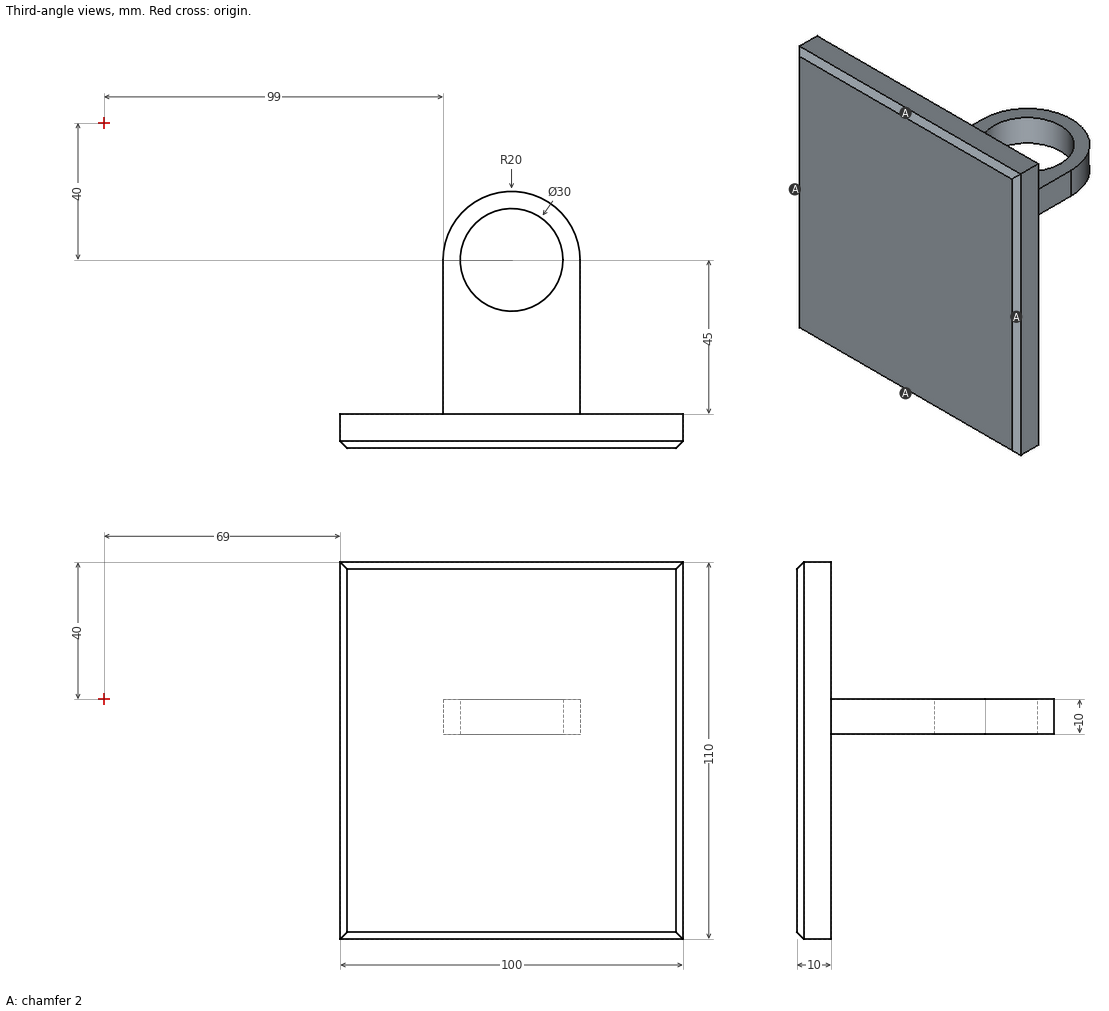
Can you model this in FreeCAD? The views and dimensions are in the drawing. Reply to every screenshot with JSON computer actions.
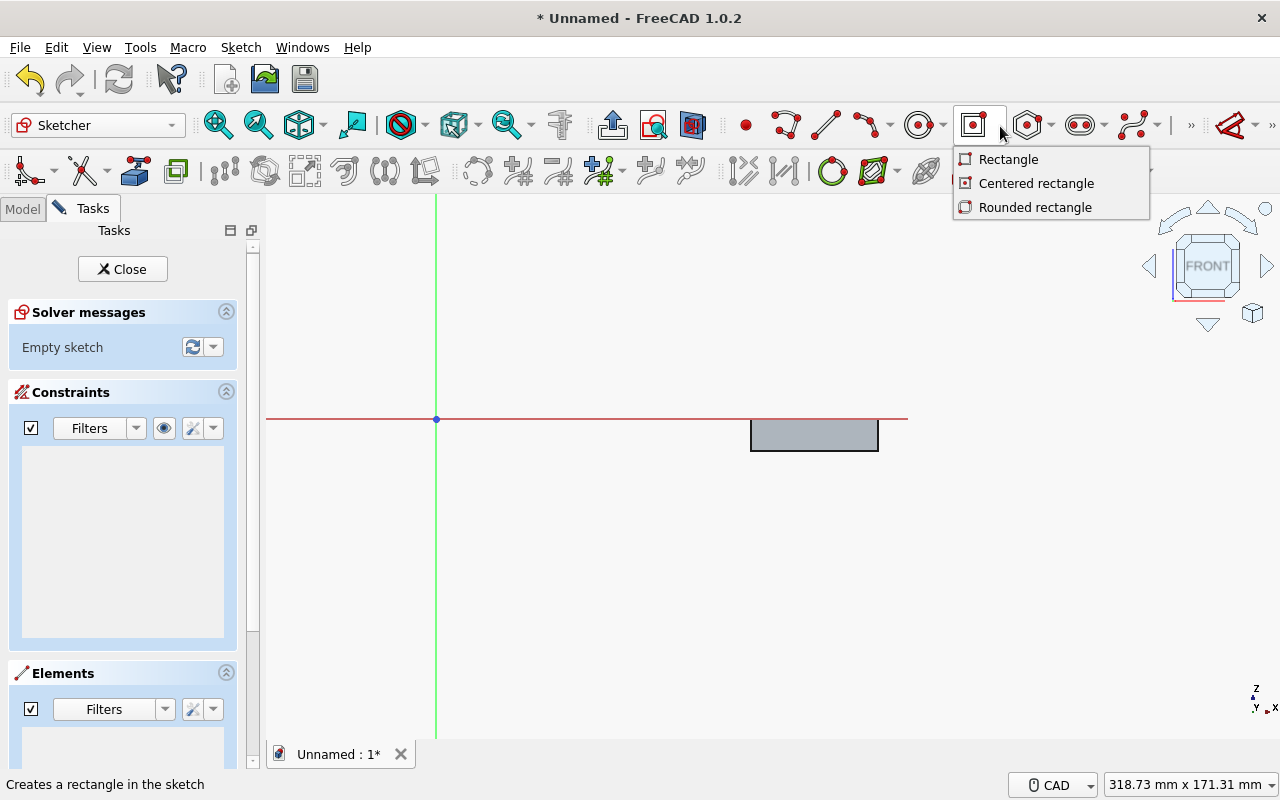
{"action": "left_click", "coordinate": [1052, 159]}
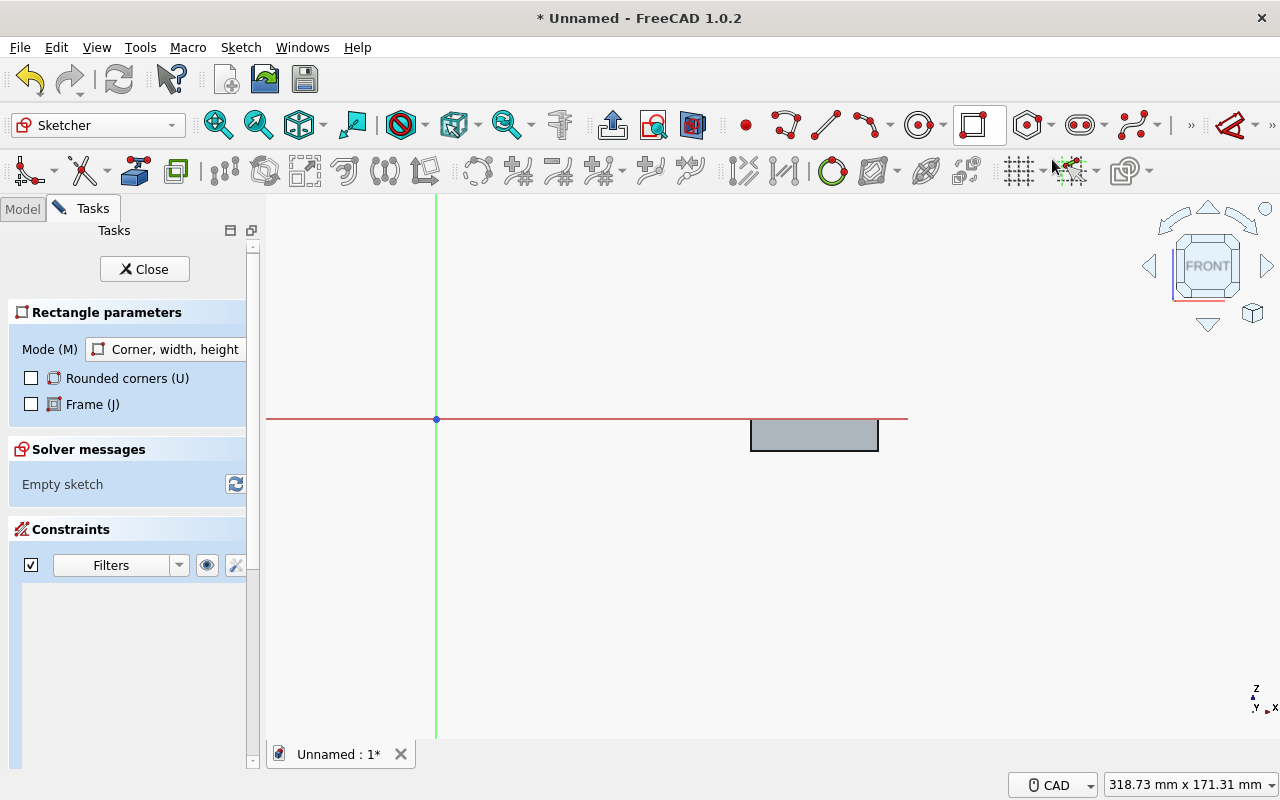
{"action": "left_click", "coordinate": [656, 292]}
{"action": "mouse_move", "coordinate": [974, 642]}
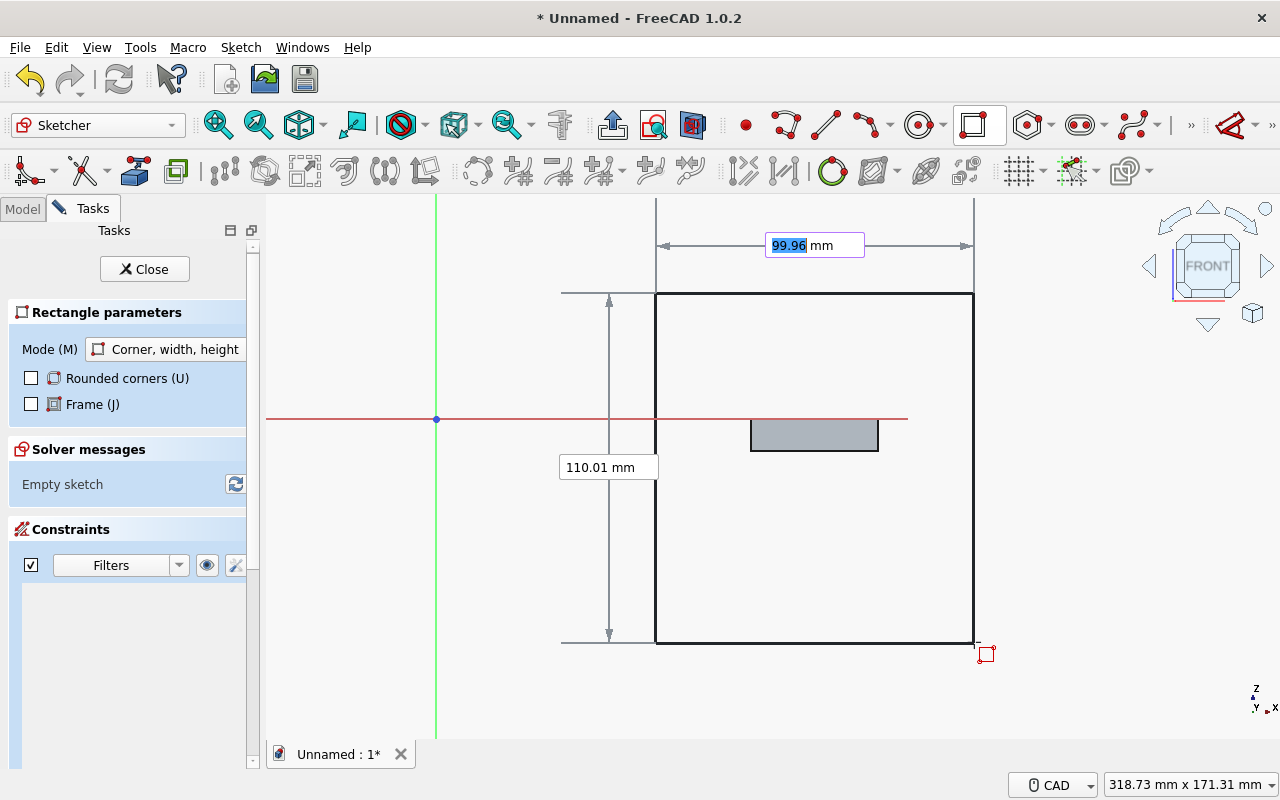
{"action": "type", "text": "100"}
{"action": "key", "text": "Tab"}
{"action": "type", "text": "110"}
{"action": "key", "text": "Return"}
{"action": "key", "text": "Escape"}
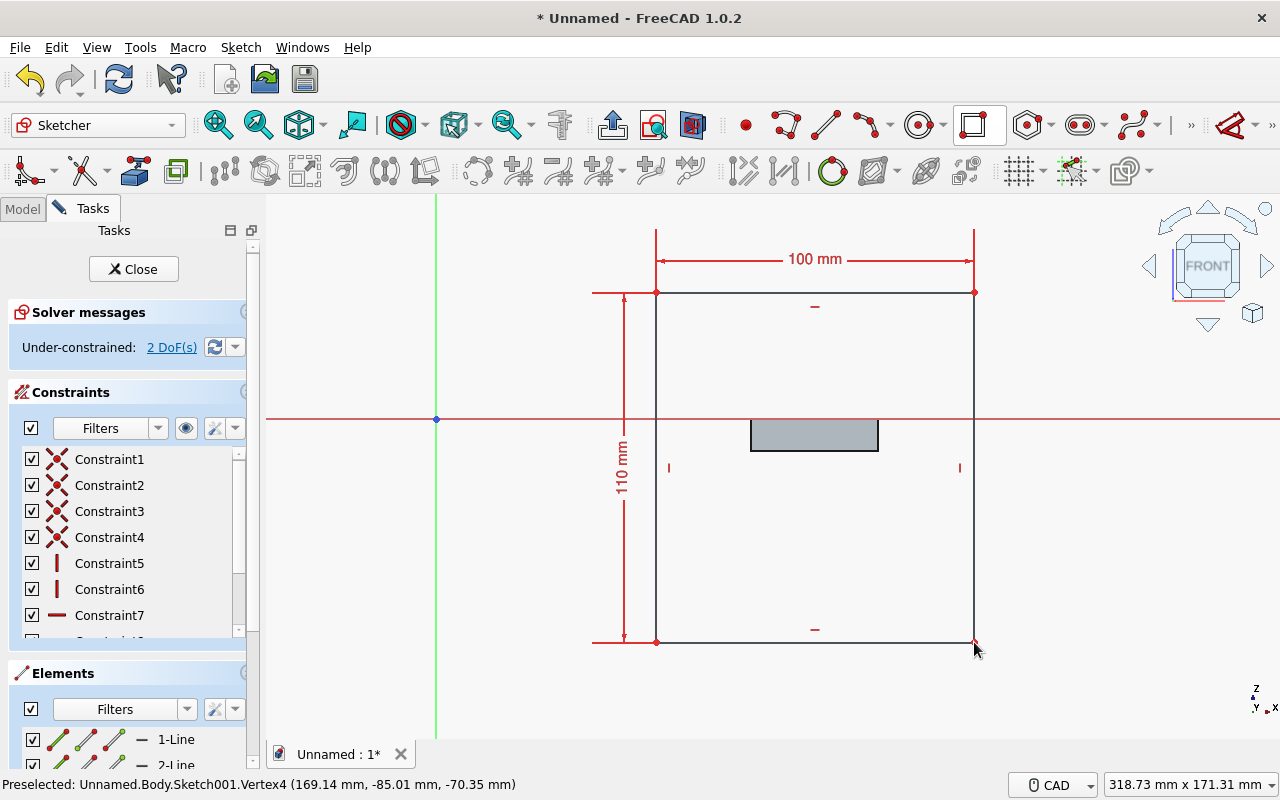
{"action": "key", "text": "d"}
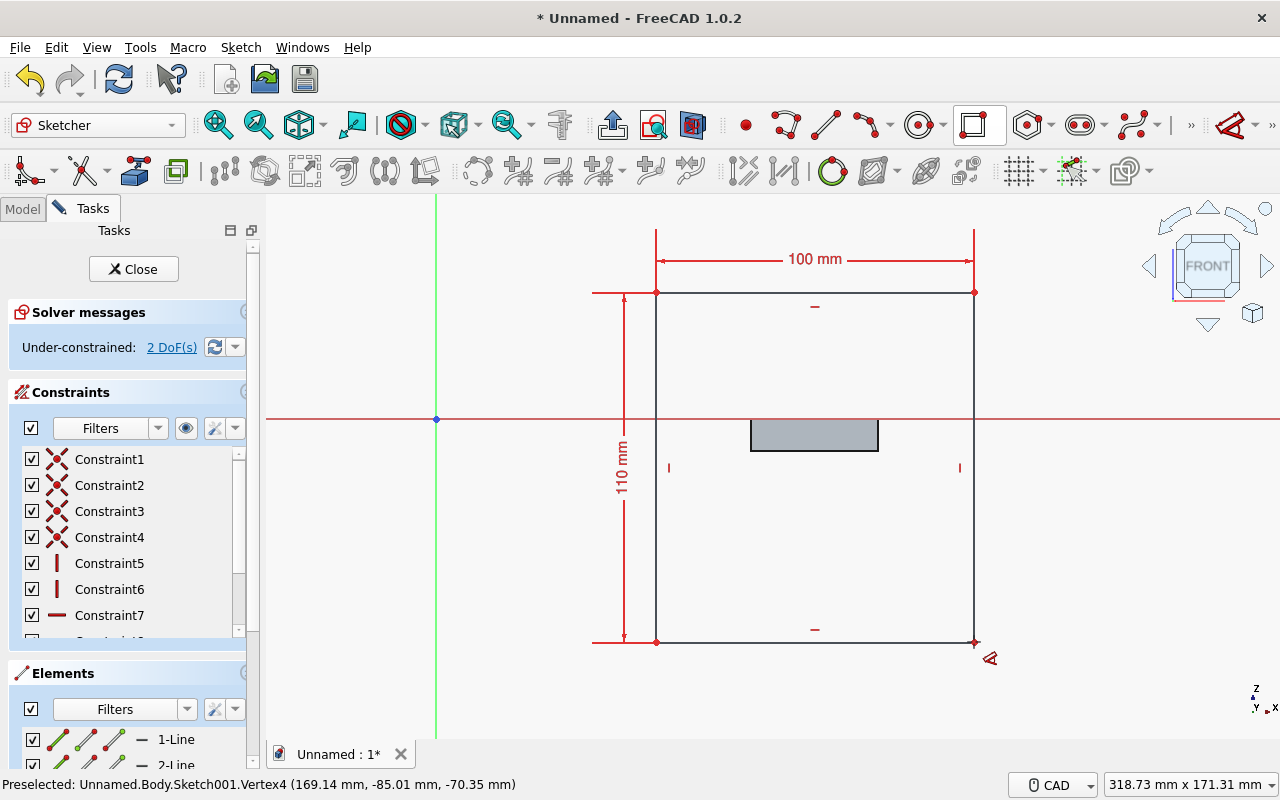
{"action": "left_click", "coordinate": [656, 293]}
{"action": "left_click", "coordinate": [546, 259]}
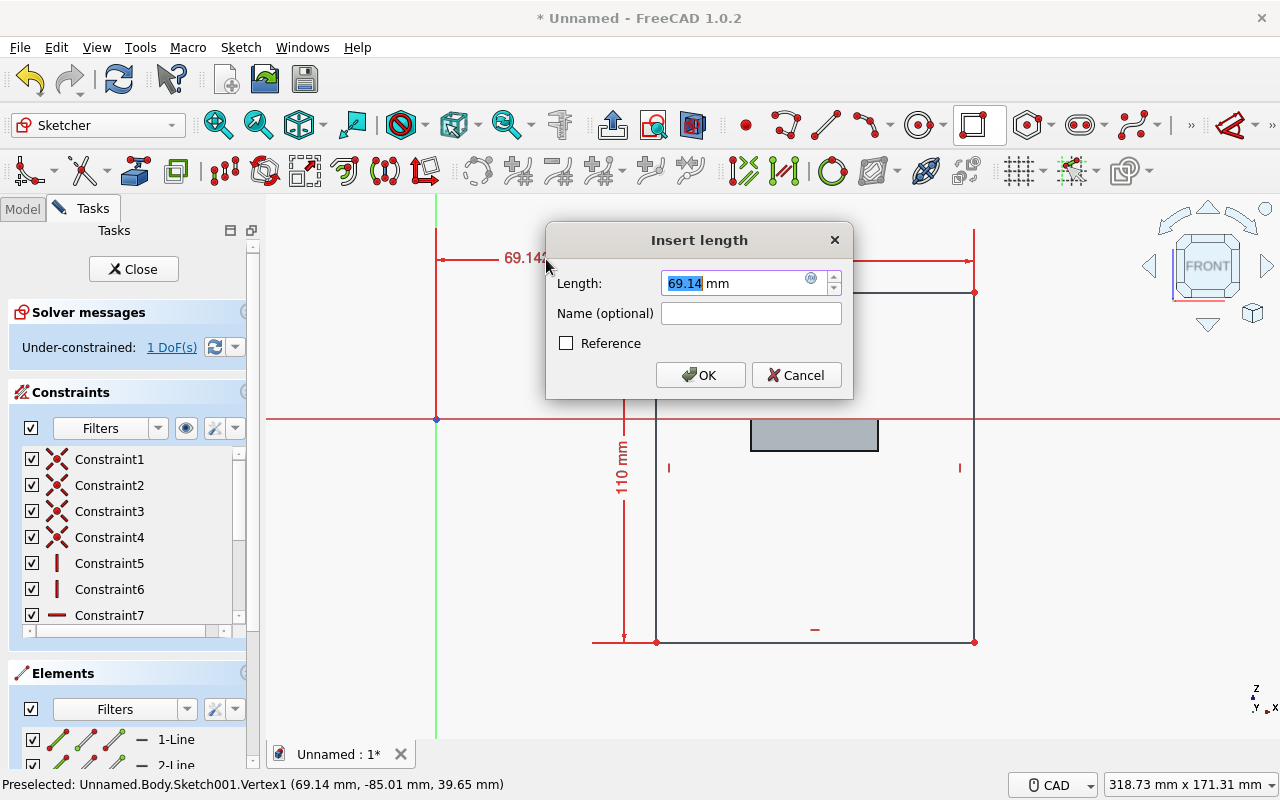
{"action": "type", "text": "69"}
{"action": "key", "text": "Return"}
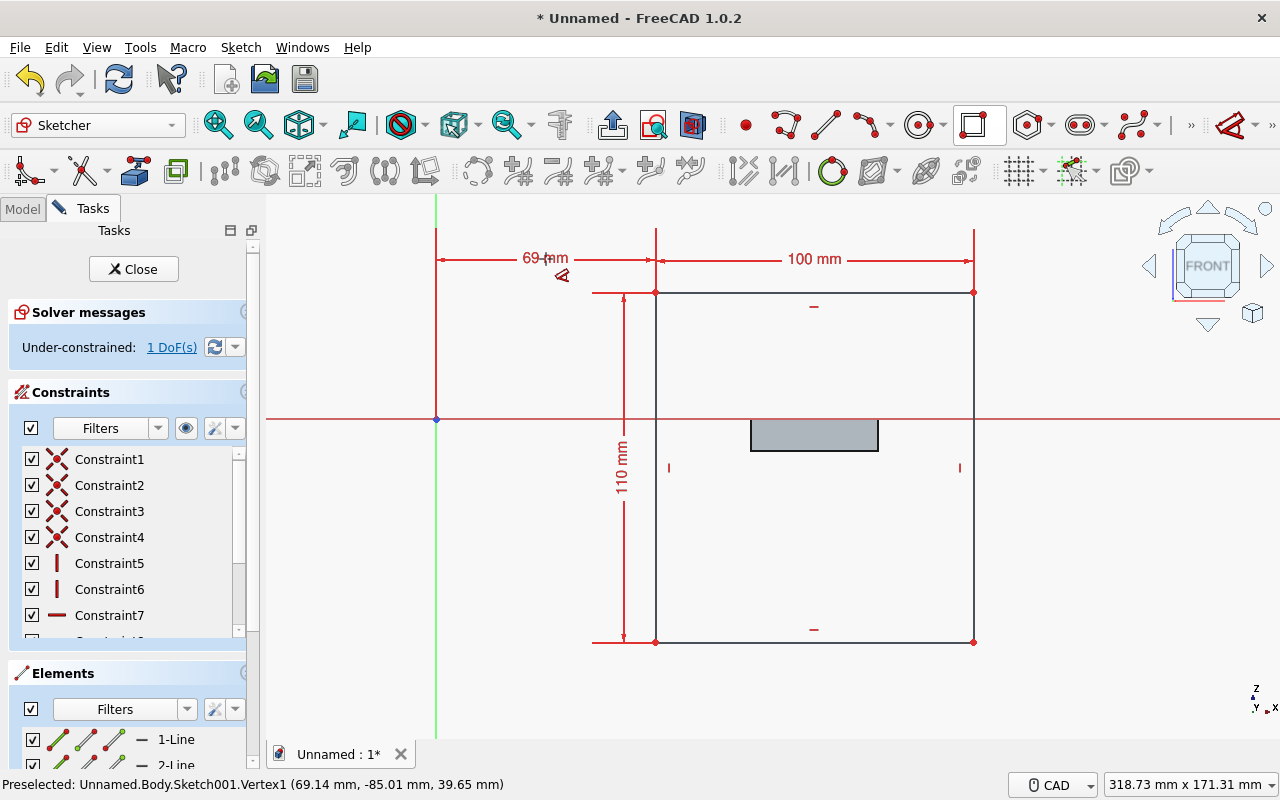
{"action": "left_click", "coordinate": [656, 293]}
{"action": "left_click", "coordinate": [402, 356]}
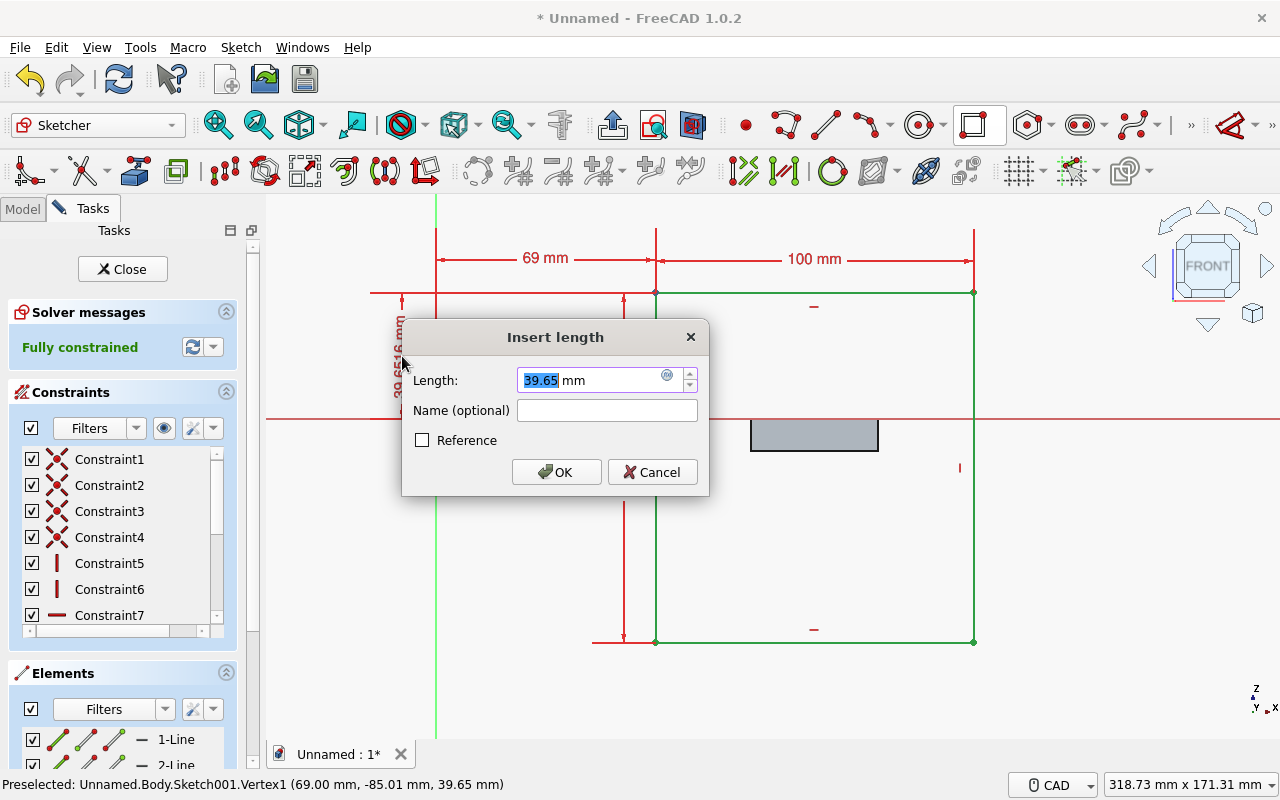
{"action": "type", "text": "40"}
{"action": "key", "text": "Return"}
{"action": "key", "text": "Escape"}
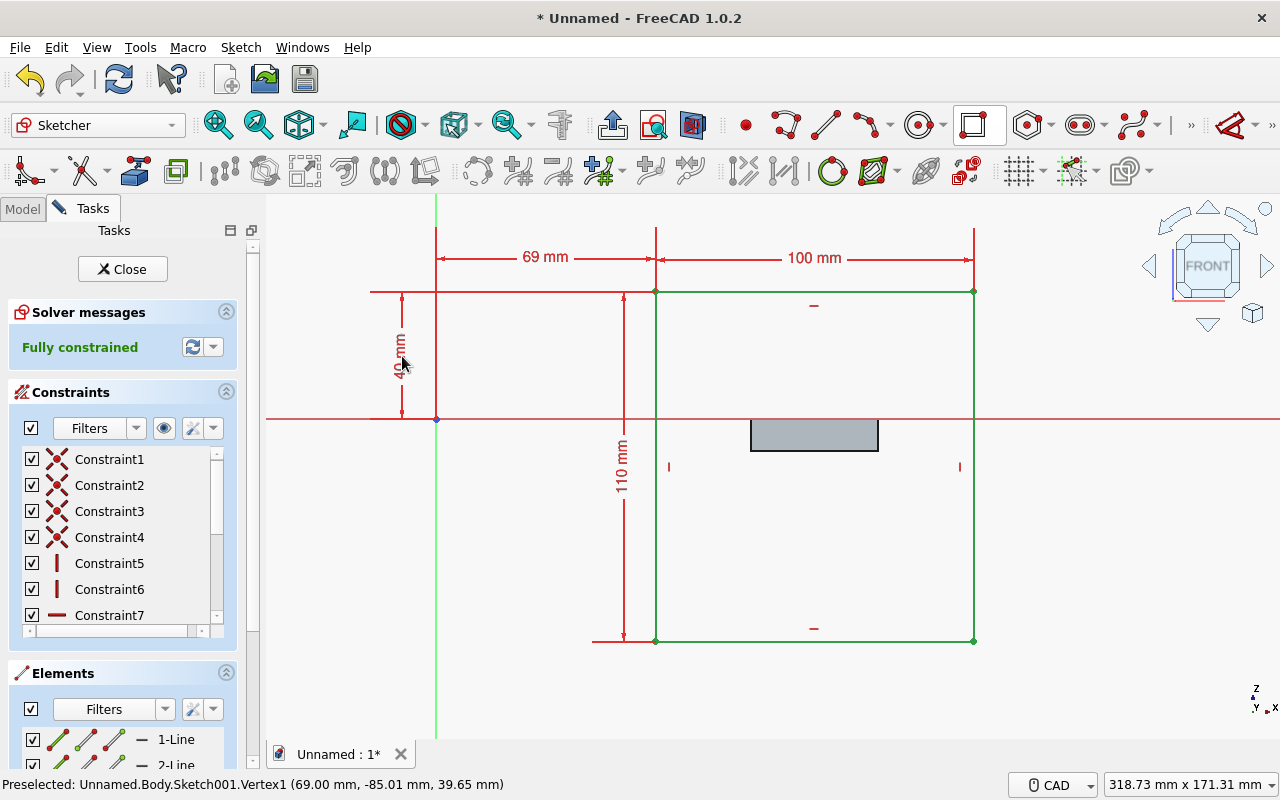
{"action": "left_click", "coordinate": [123, 269]}